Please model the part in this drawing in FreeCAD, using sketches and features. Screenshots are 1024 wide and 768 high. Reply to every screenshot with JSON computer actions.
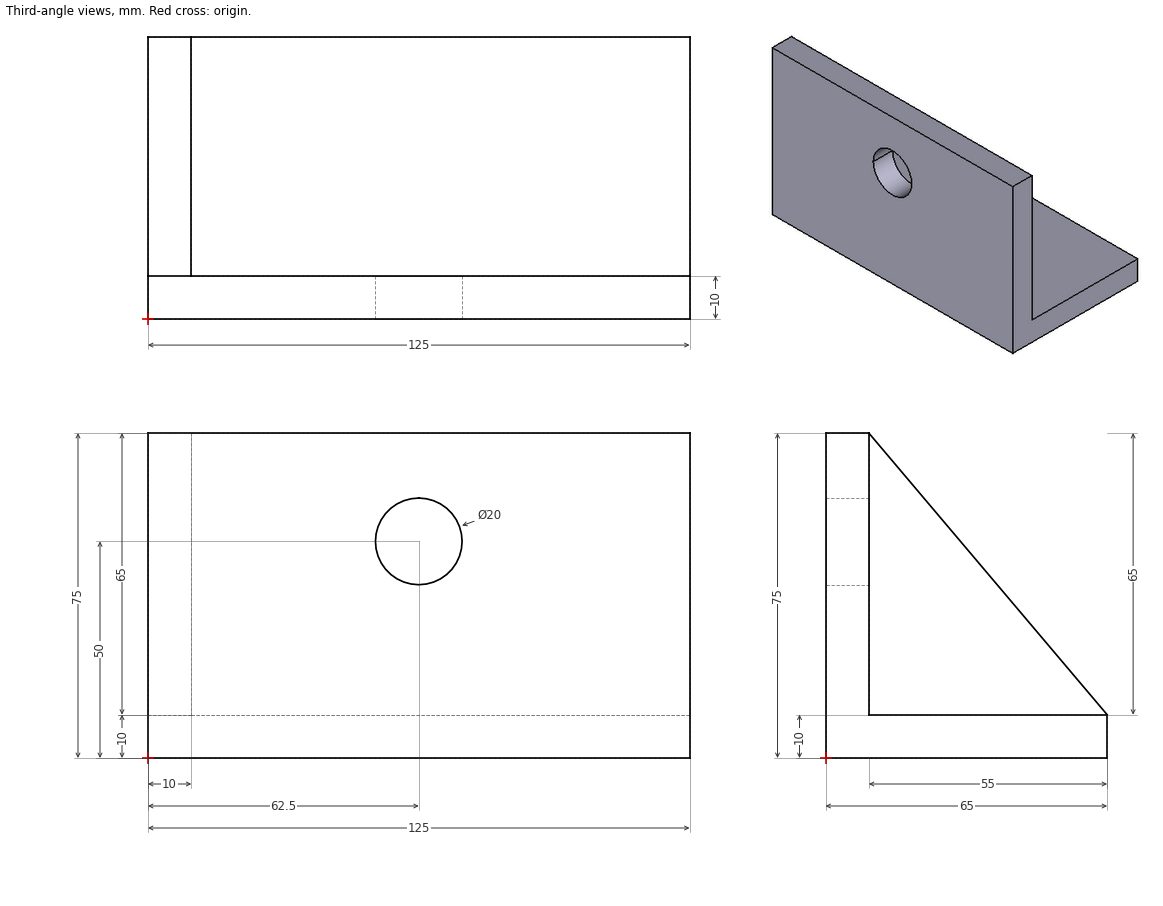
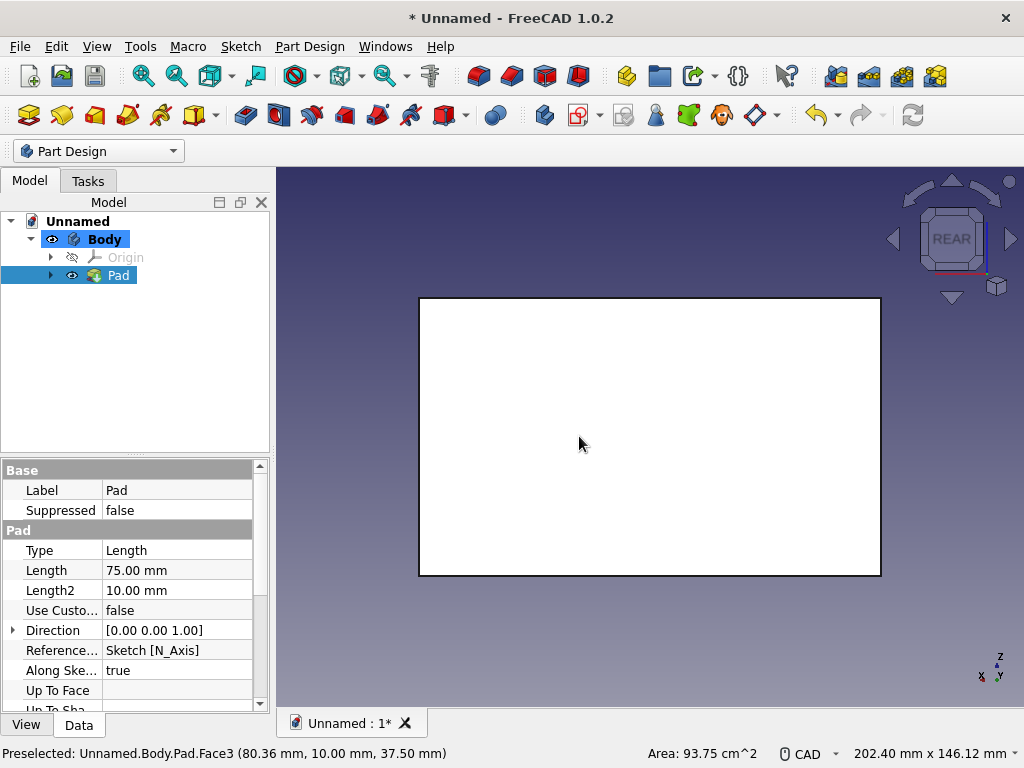
{"action": "left_click", "coordinate": [578, 116]}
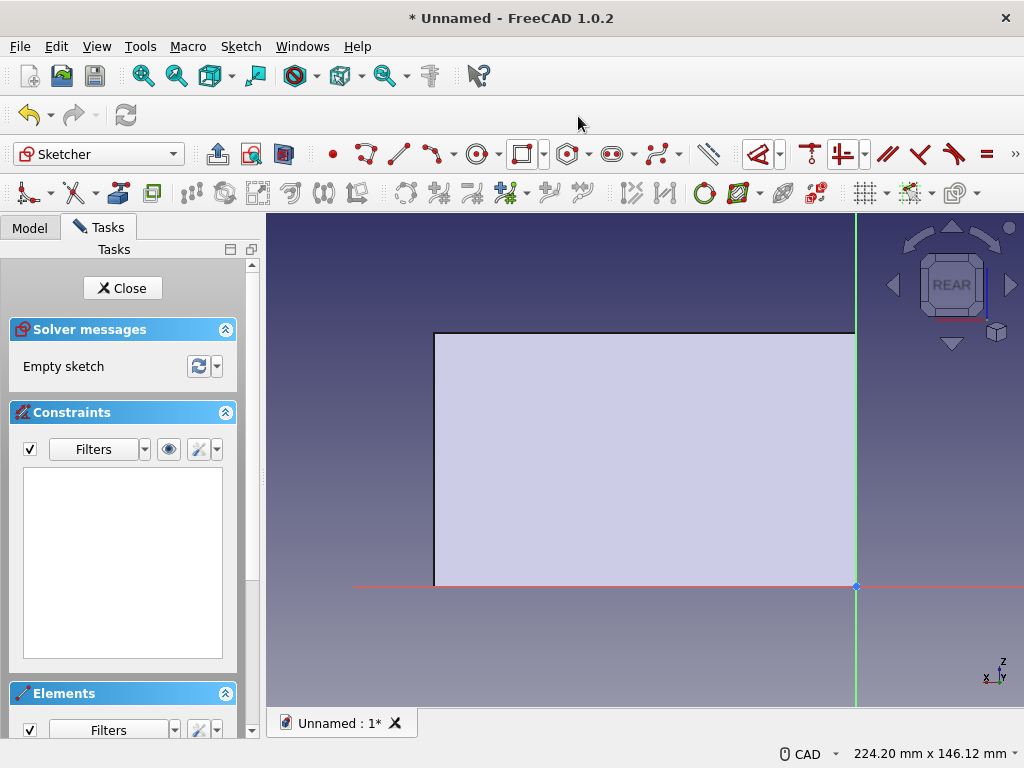
{"action": "scroll", "coordinate": [294, 241], "scroll_direction": "down", "scroll_amount": 1}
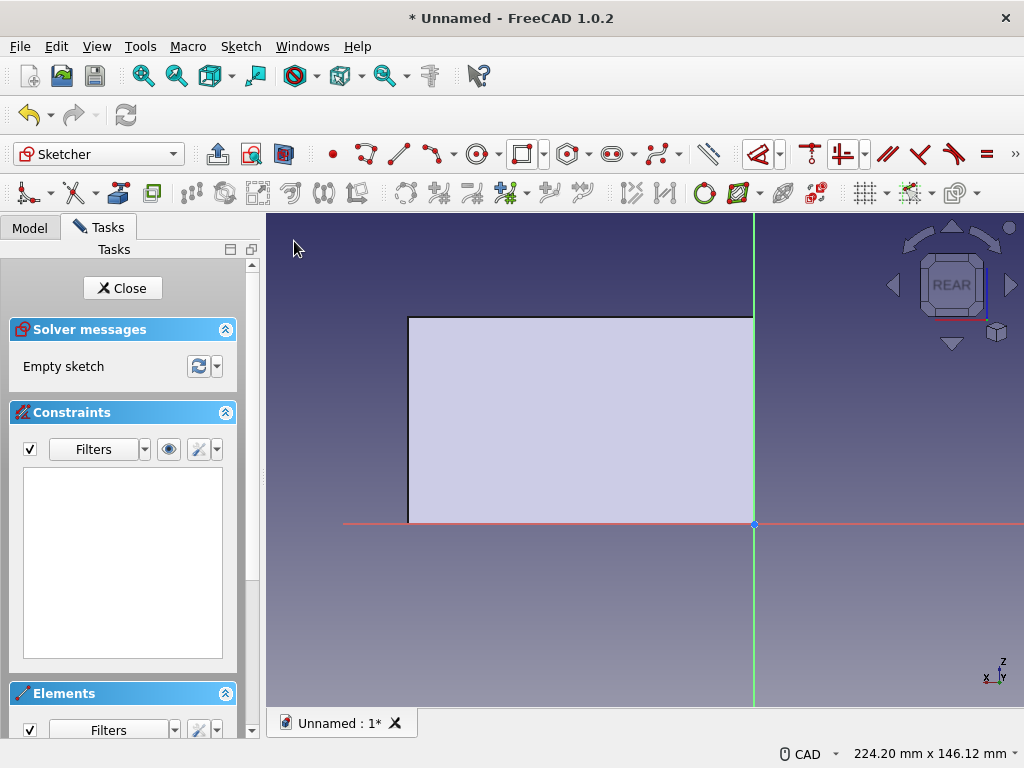
{"action": "key", "text": "g r"}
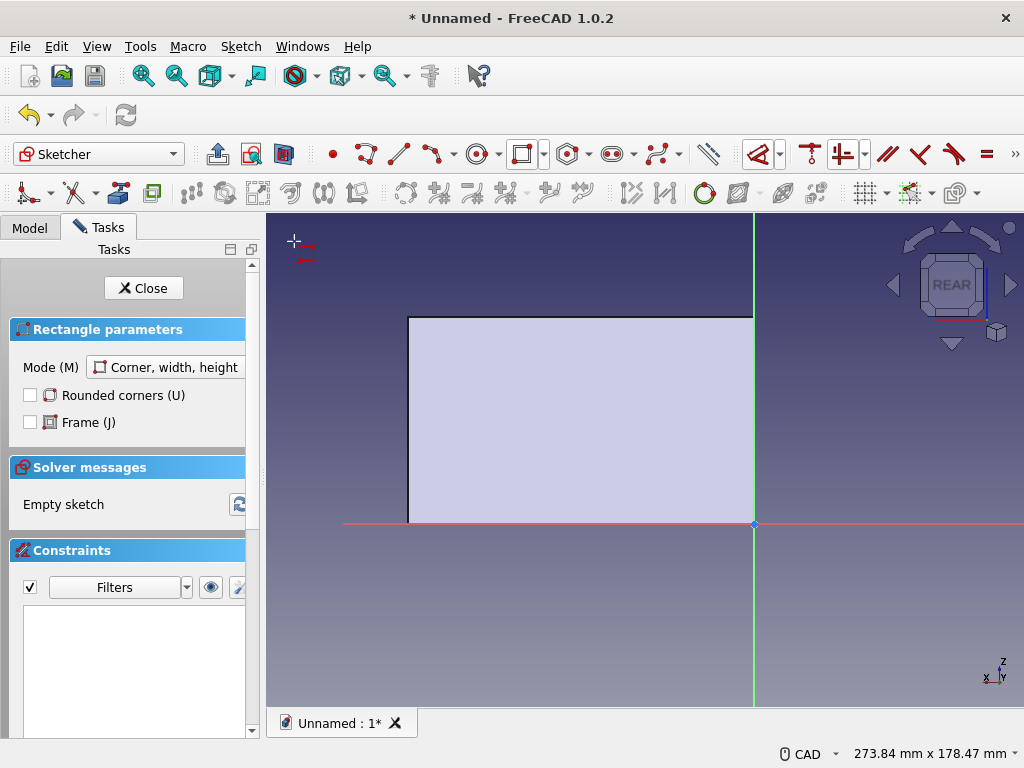
{"action": "left_click", "coordinate": [754, 524]}
{"action": "left_click", "coordinate": [408, 496]}
{"action": "key", "text": "Escape"}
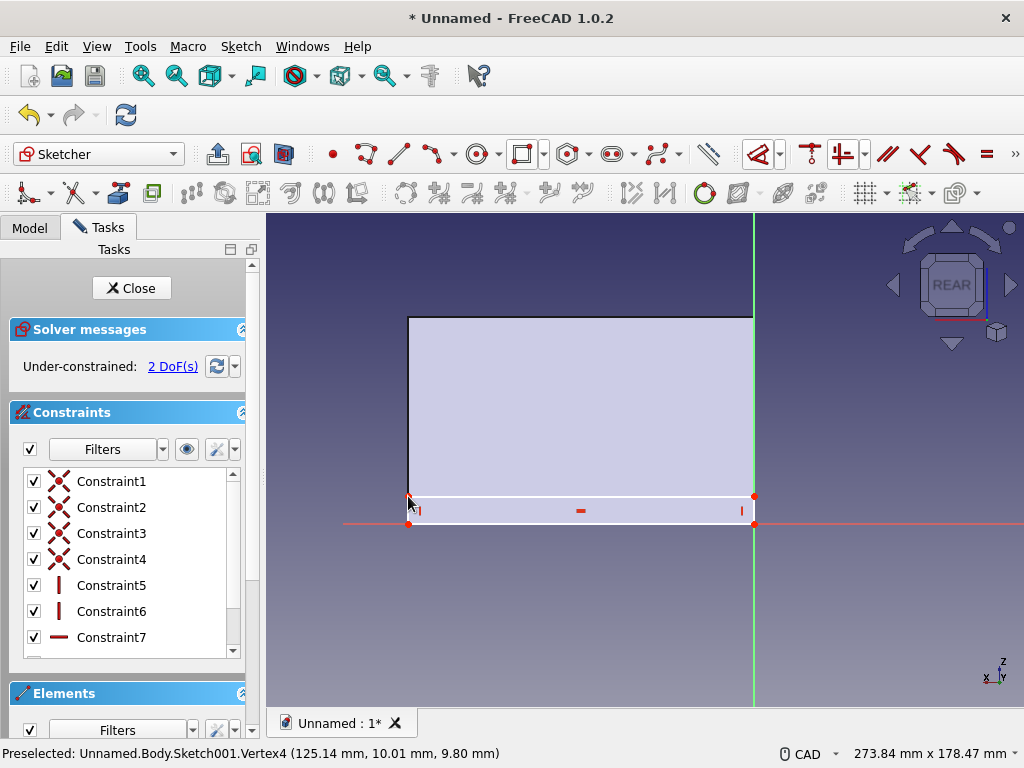
{"action": "scroll", "coordinate": [754, 513], "scroll_direction": "up", "scroll_amount": 2}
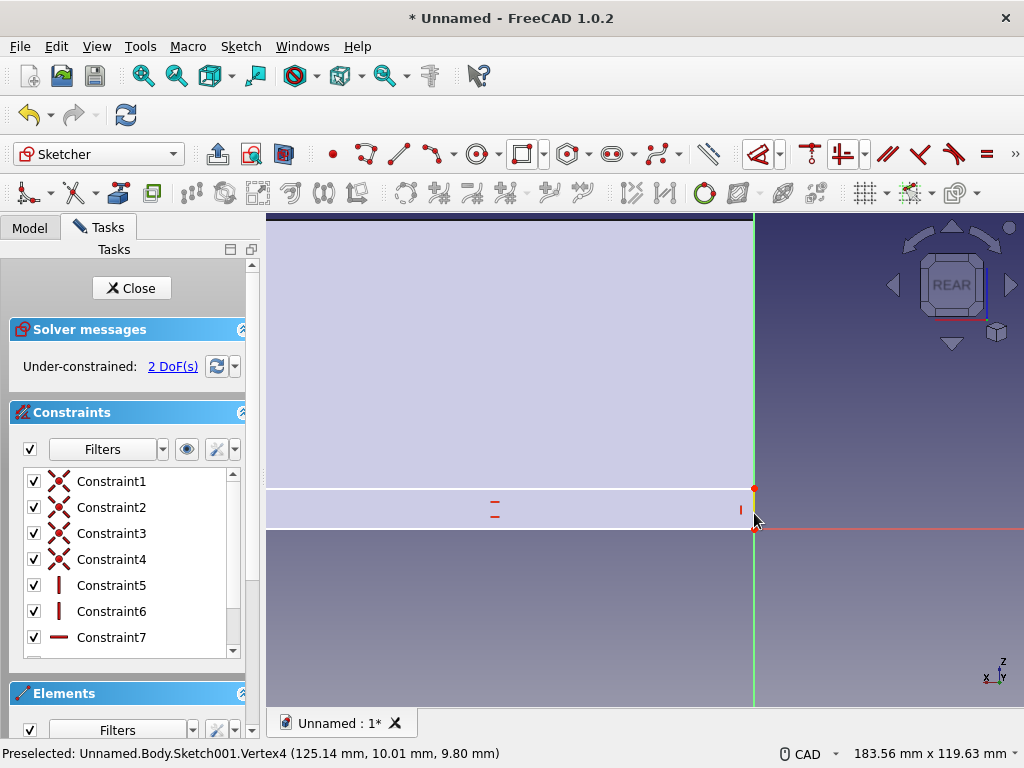
{"action": "left_click", "coordinate": [754, 513]}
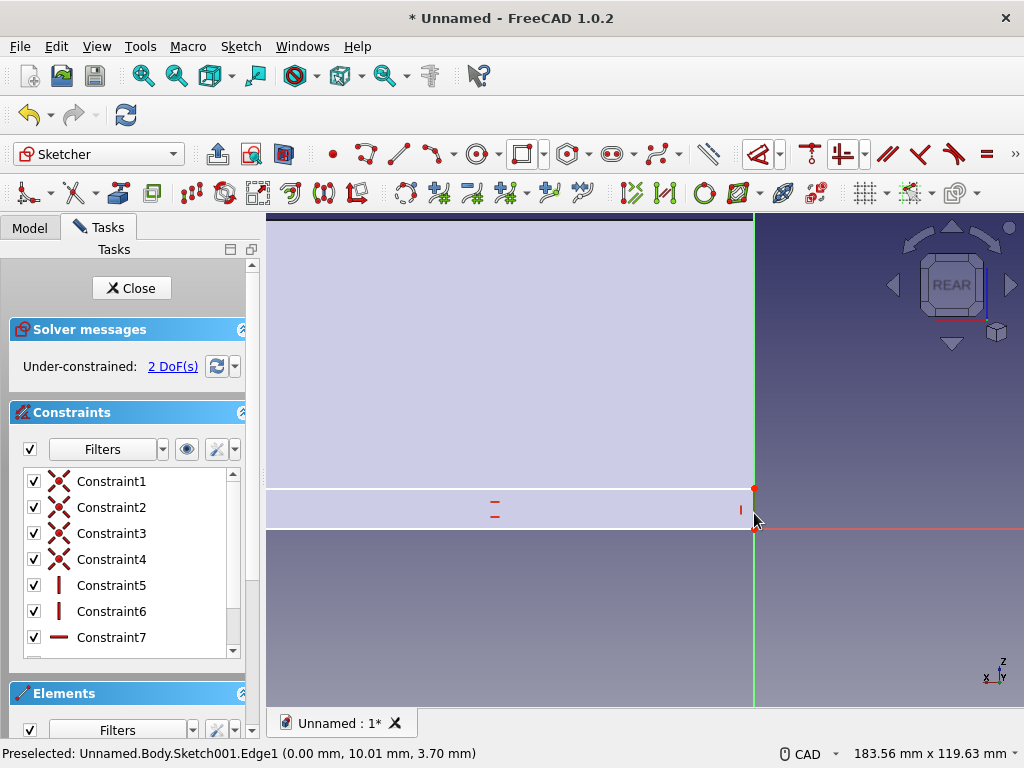
{"action": "left_click", "coordinate": [780, 154]}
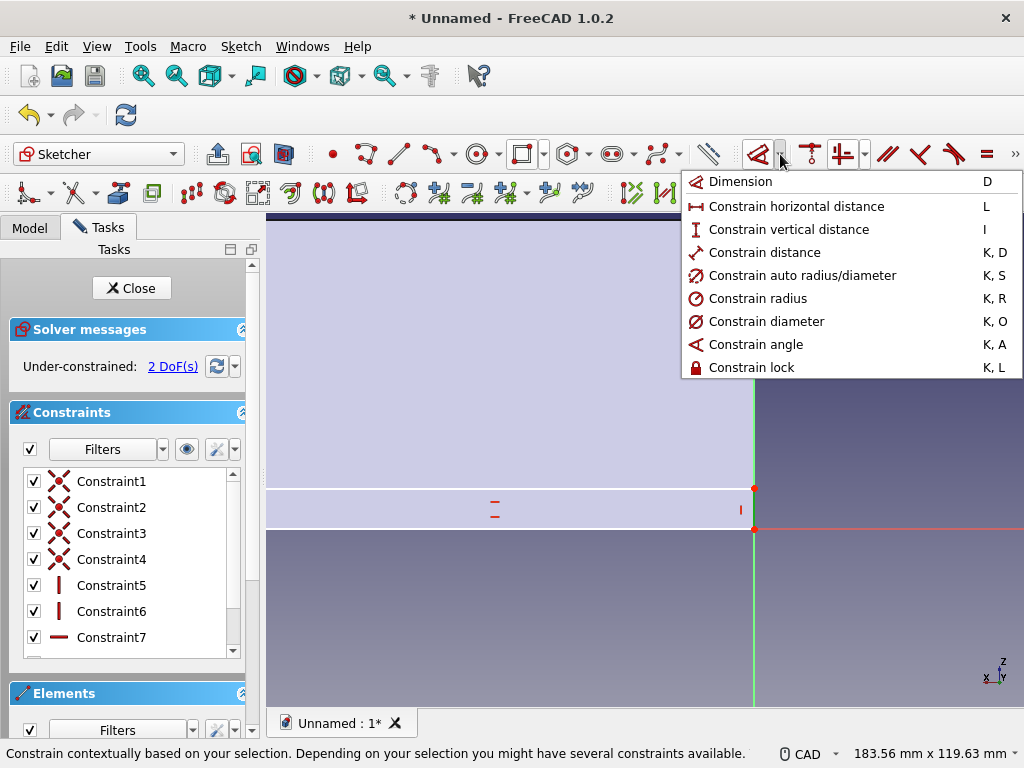
{"action": "left_click", "coordinate": [852, 230]}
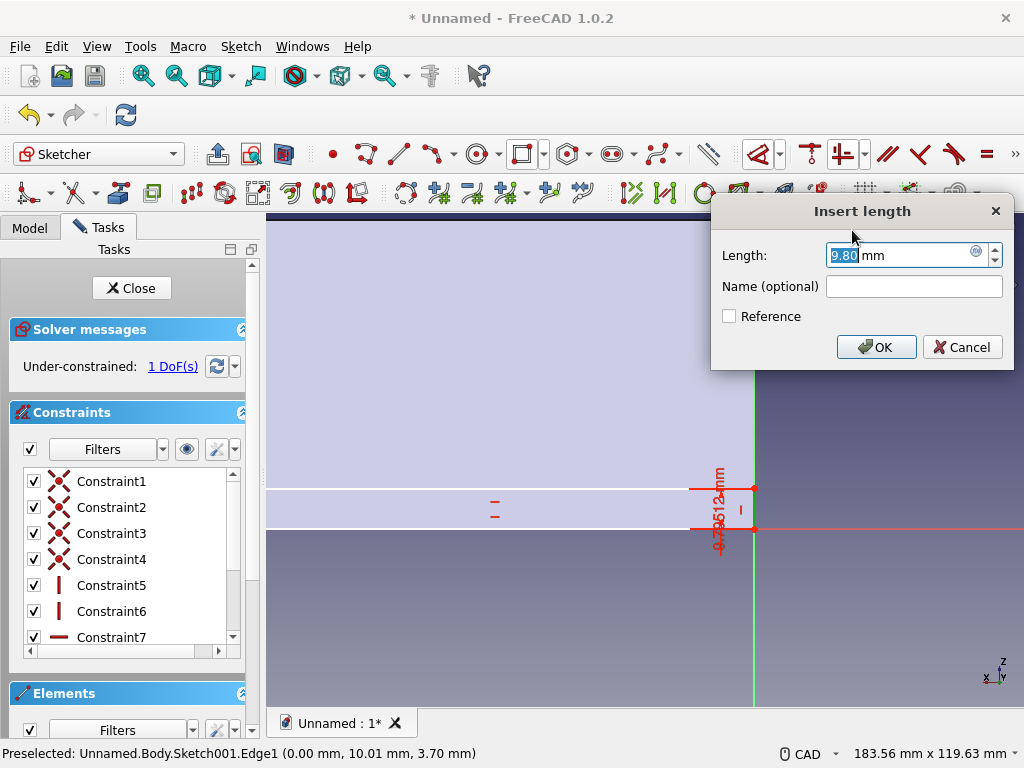
{"action": "type", "text": "10"}
{"action": "key", "text": "Return"}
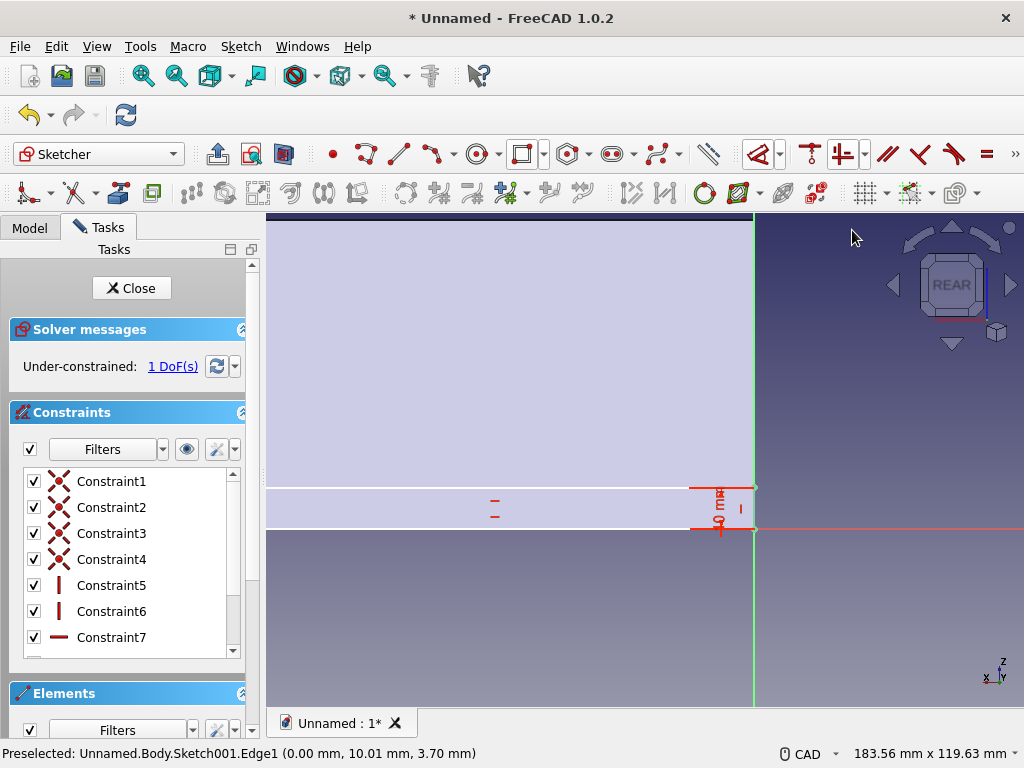
{"action": "left_click", "coordinate": [599, 488]}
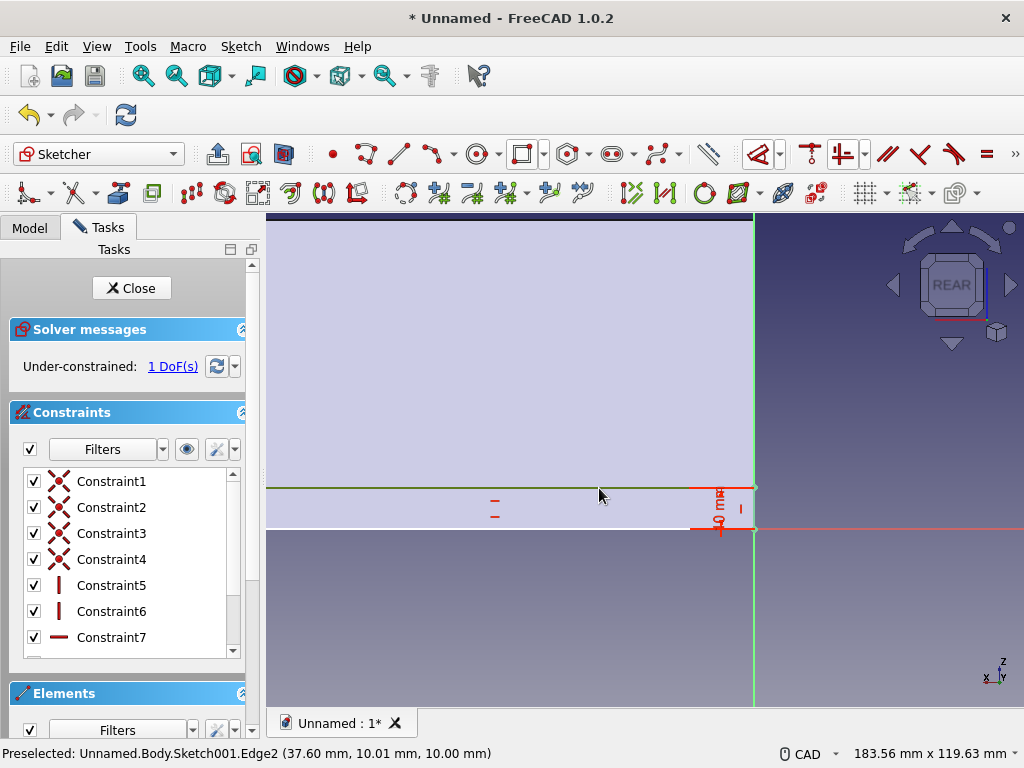
{"action": "key", "text": "l"}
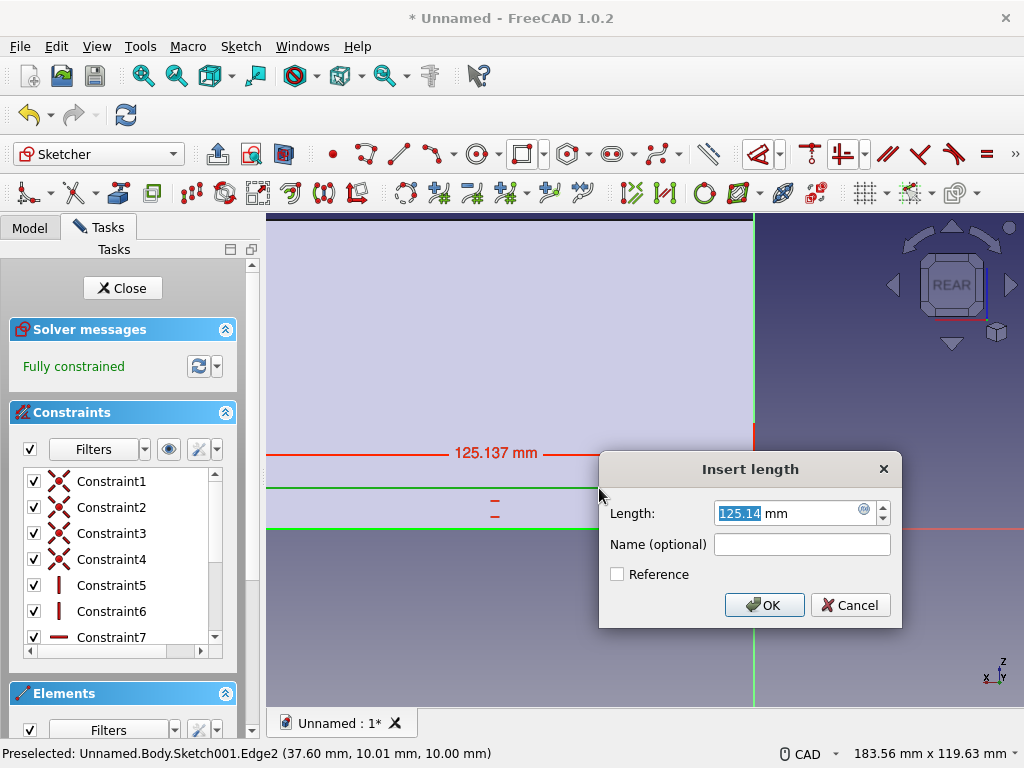
{"action": "type", "text": "125"}
{"action": "key", "text": "Return"}